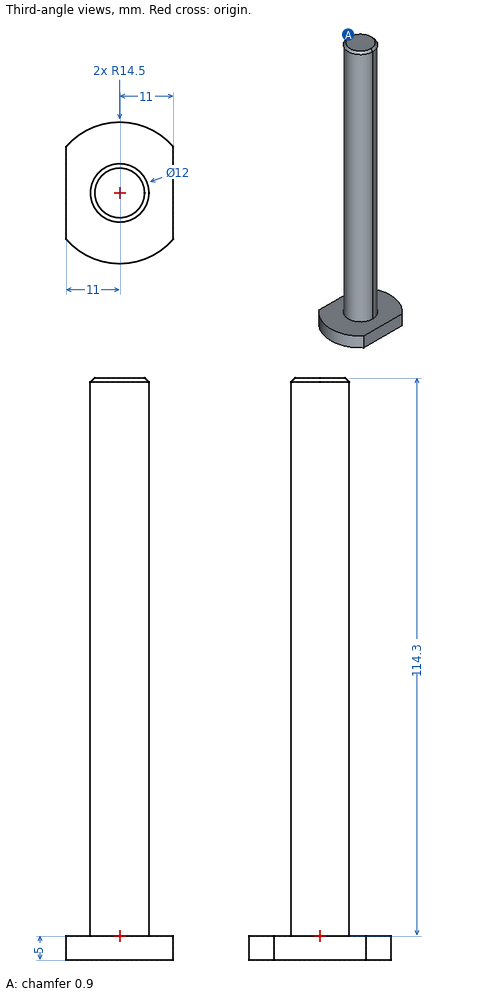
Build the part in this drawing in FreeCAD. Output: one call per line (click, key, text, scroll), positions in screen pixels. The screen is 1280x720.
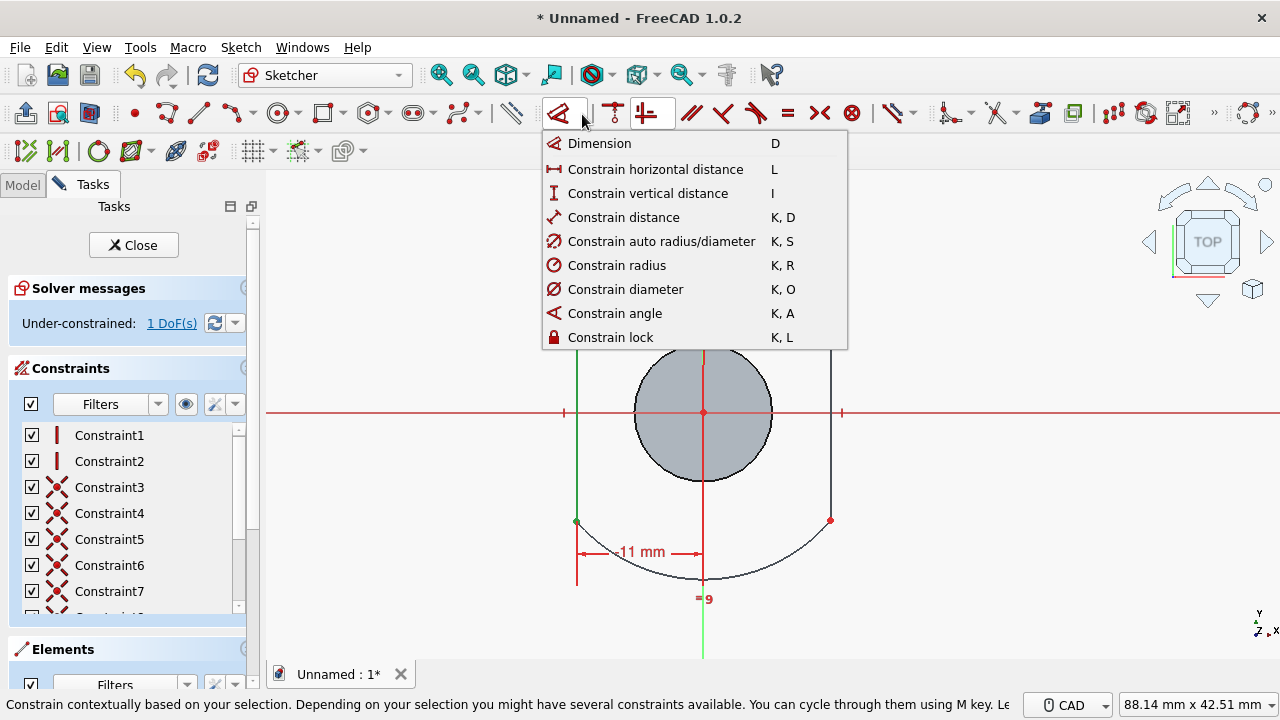
click(695, 169)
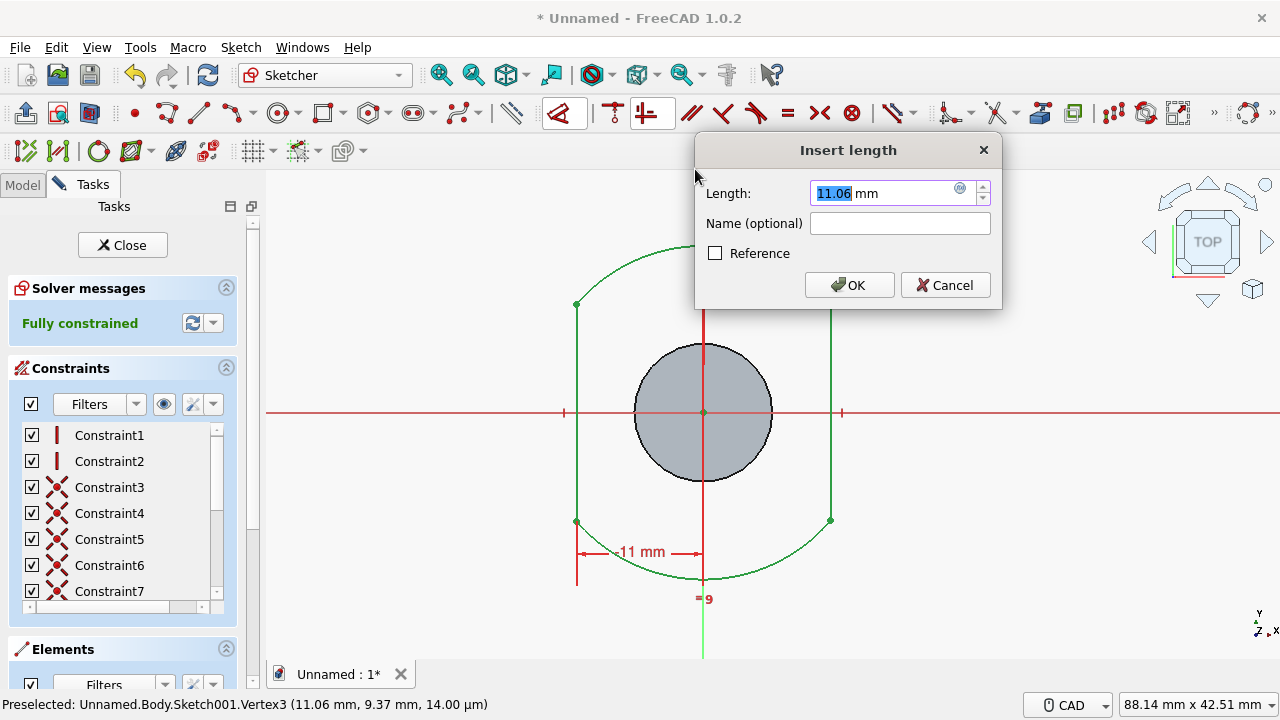
text(11)
key(Return)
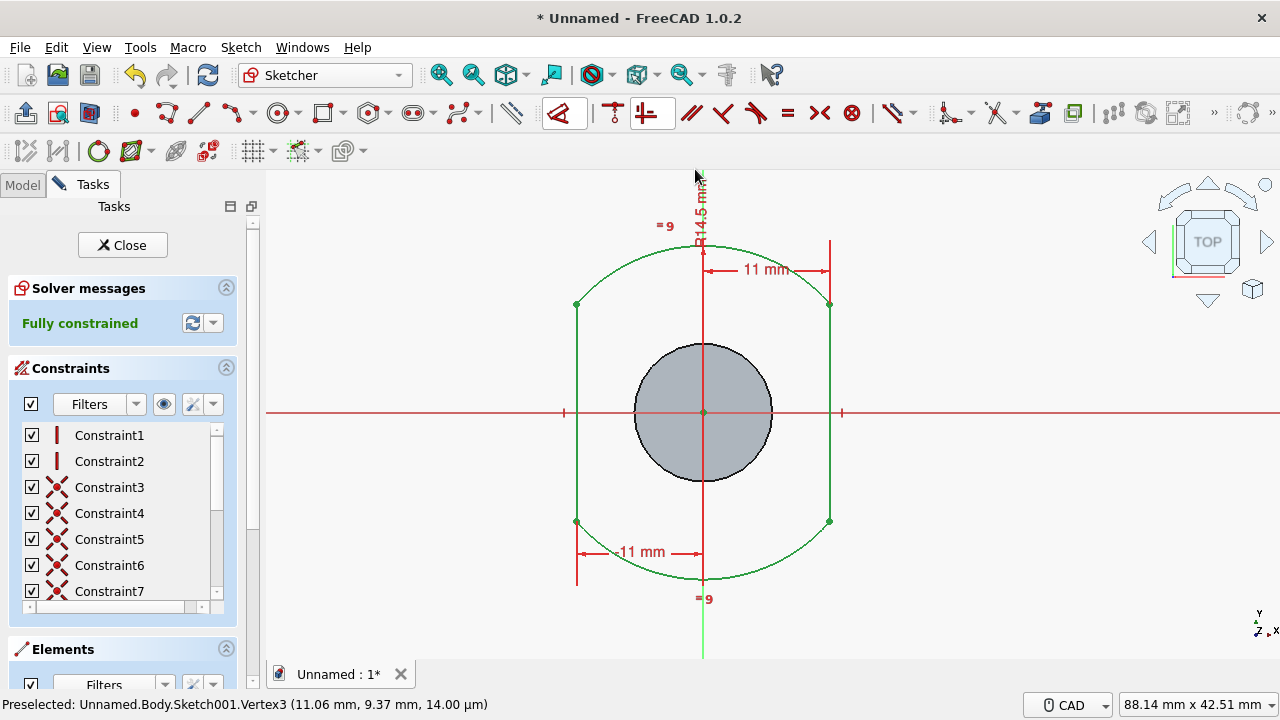
click(123, 245)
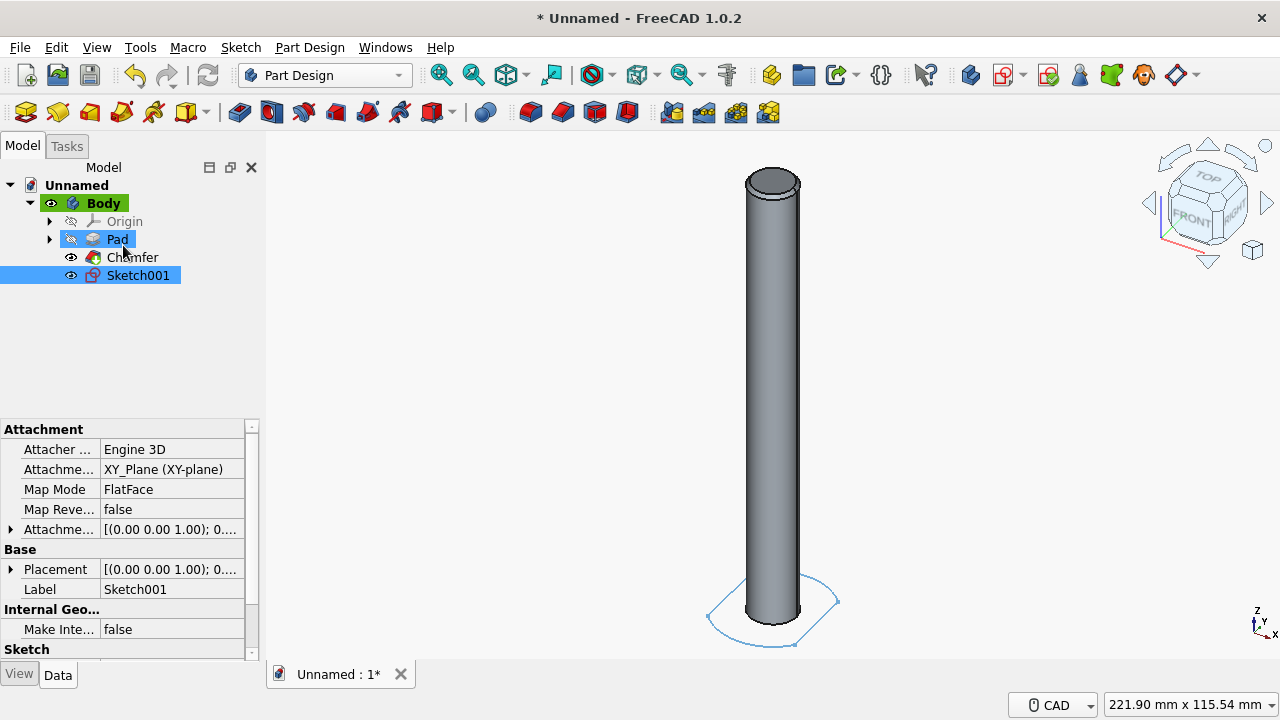
click(26, 112)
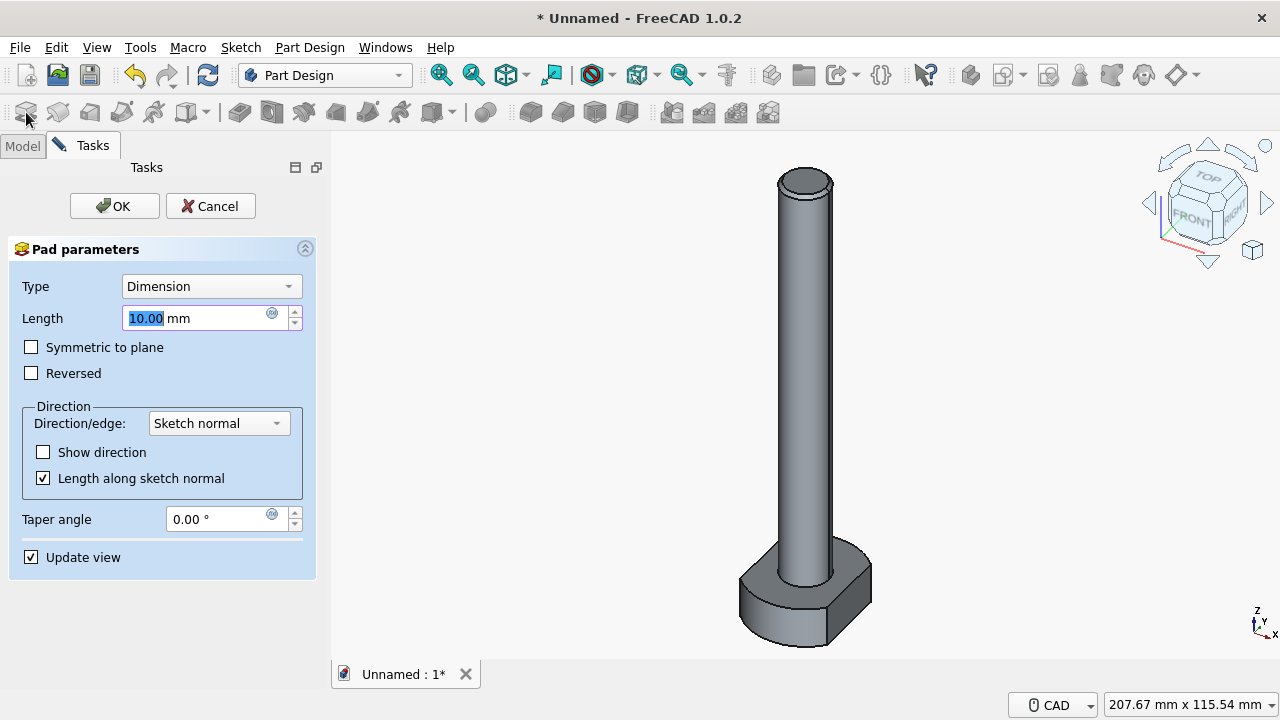
text(5)
key(Tab)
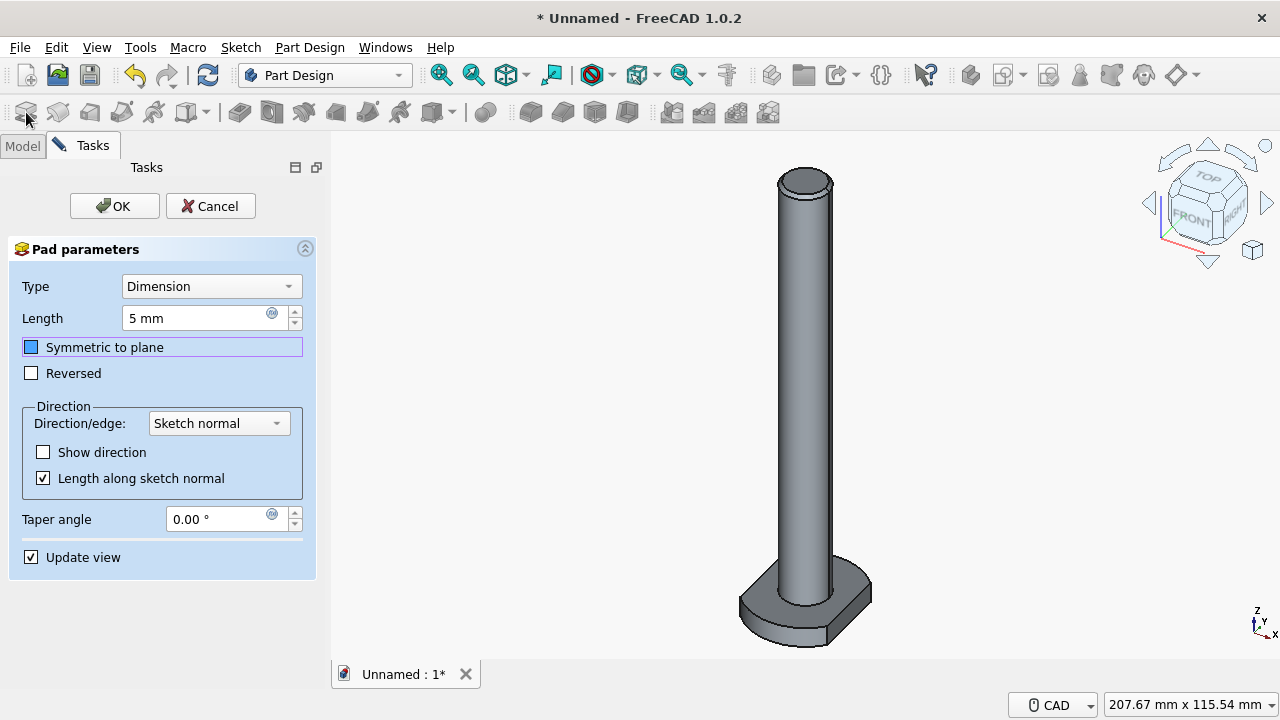
click(30, 373)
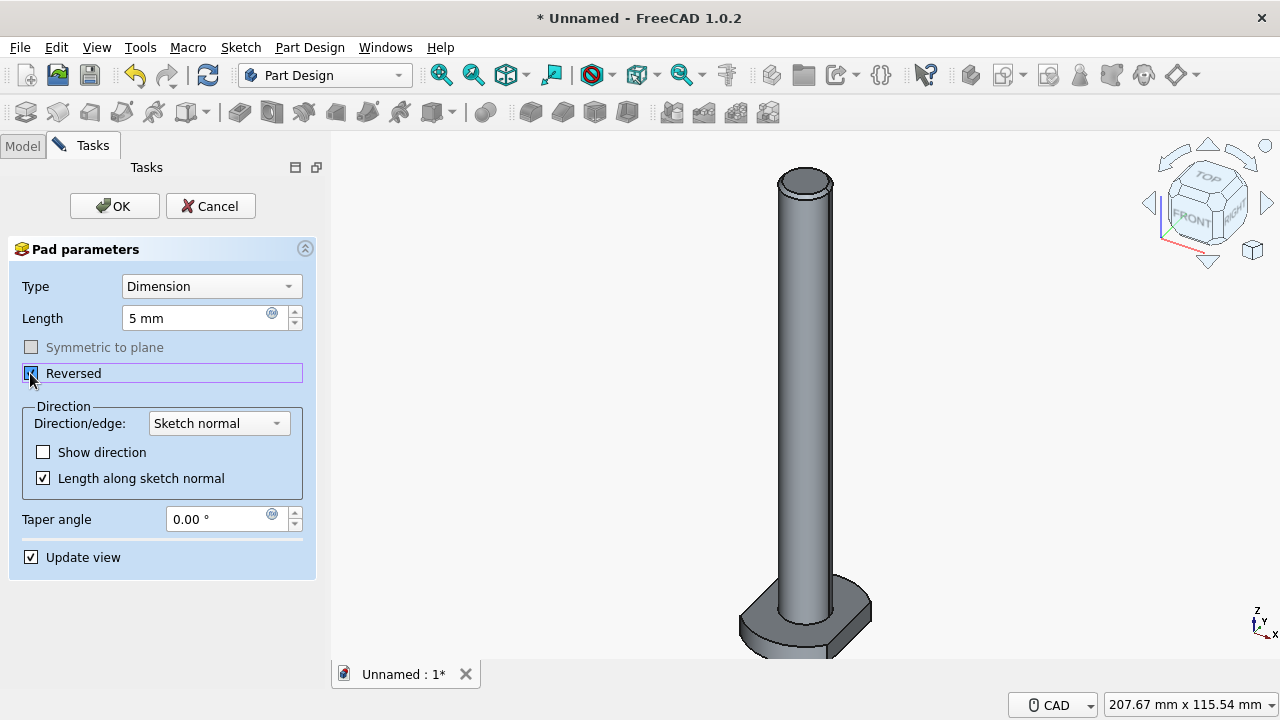
click(115, 206)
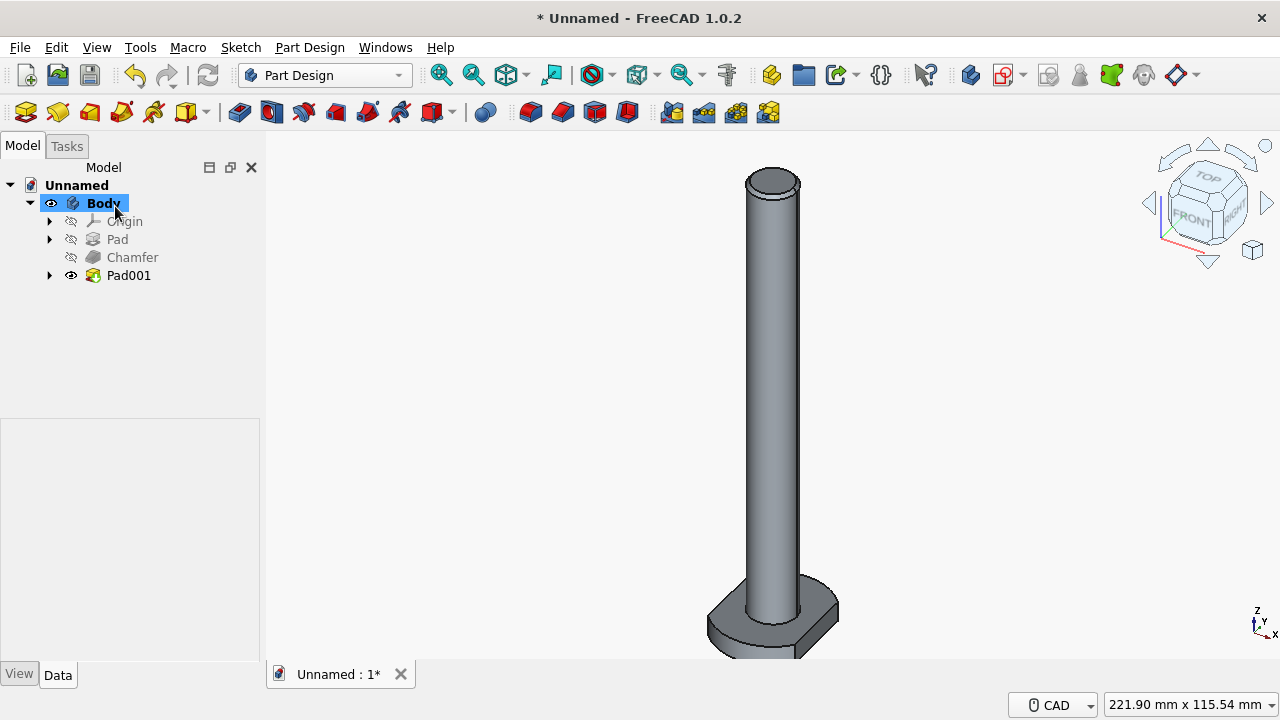
key(0)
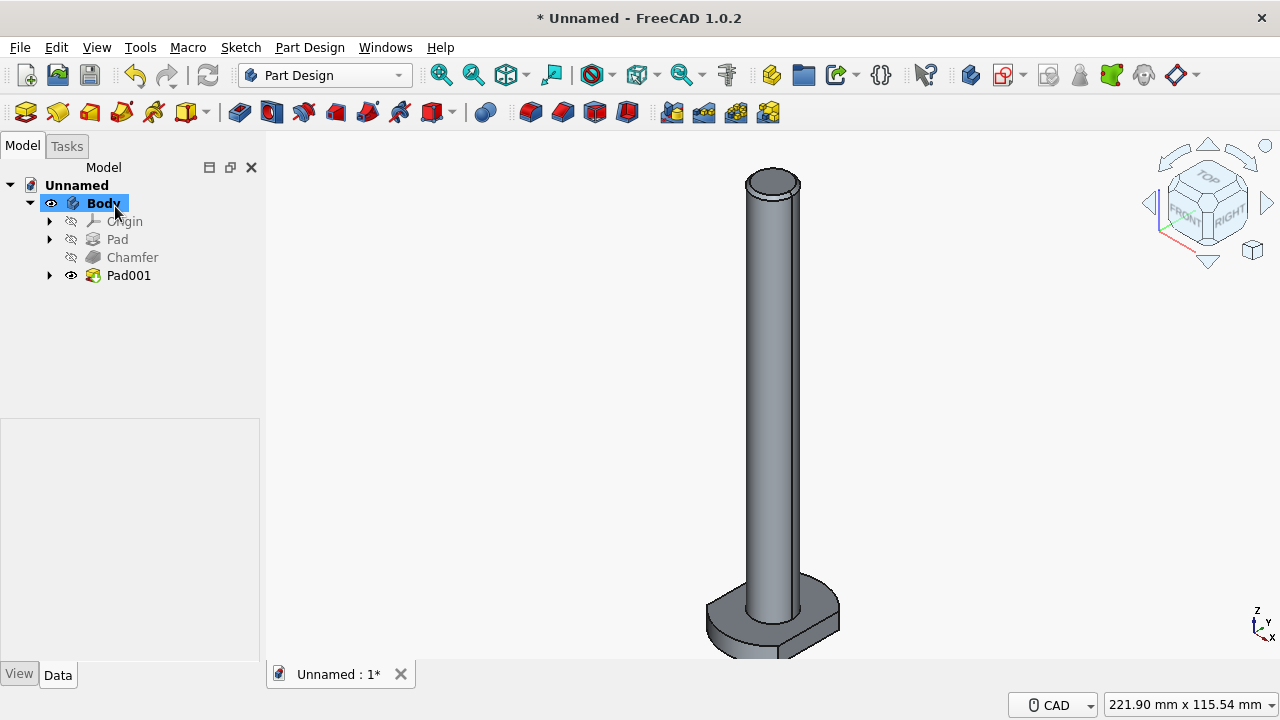
click(442, 76)